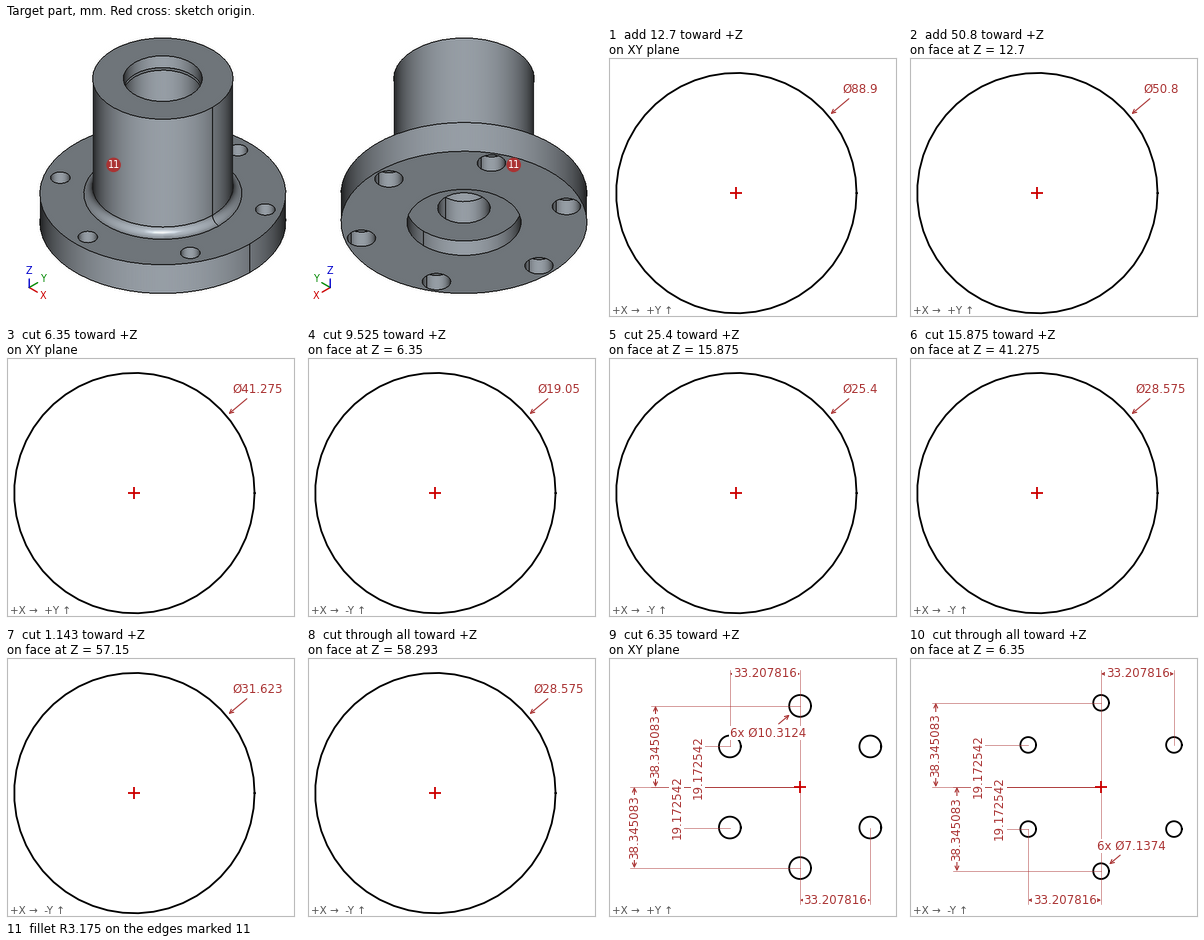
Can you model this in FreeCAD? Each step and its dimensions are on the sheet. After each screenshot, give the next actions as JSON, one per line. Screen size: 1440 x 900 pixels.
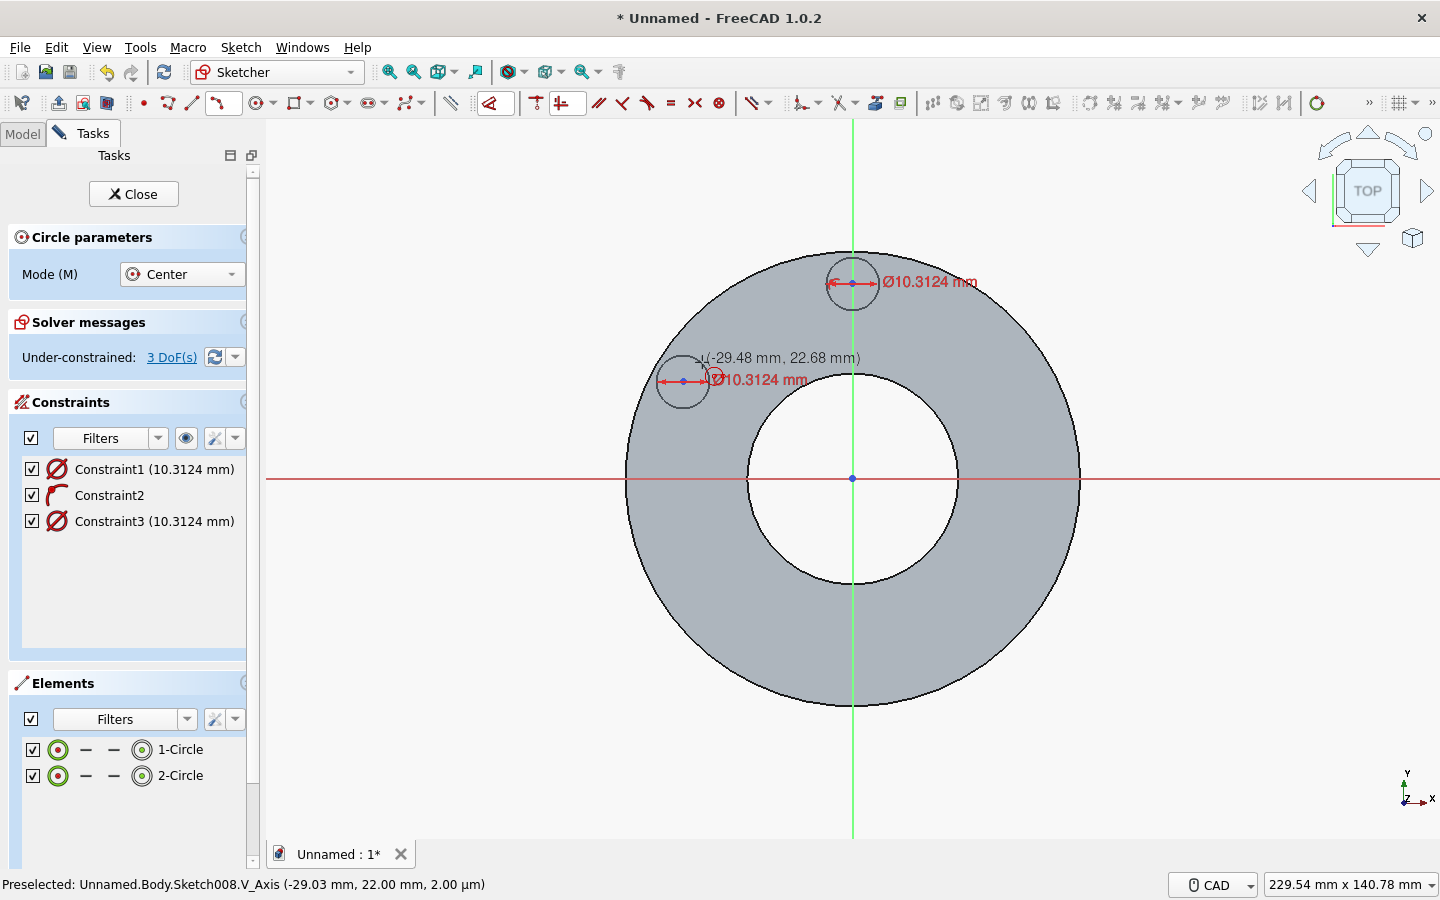
{"action": "left_click", "coordinate": [683, 577]}
{"action": "mouse_move", "coordinate": [702, 558]}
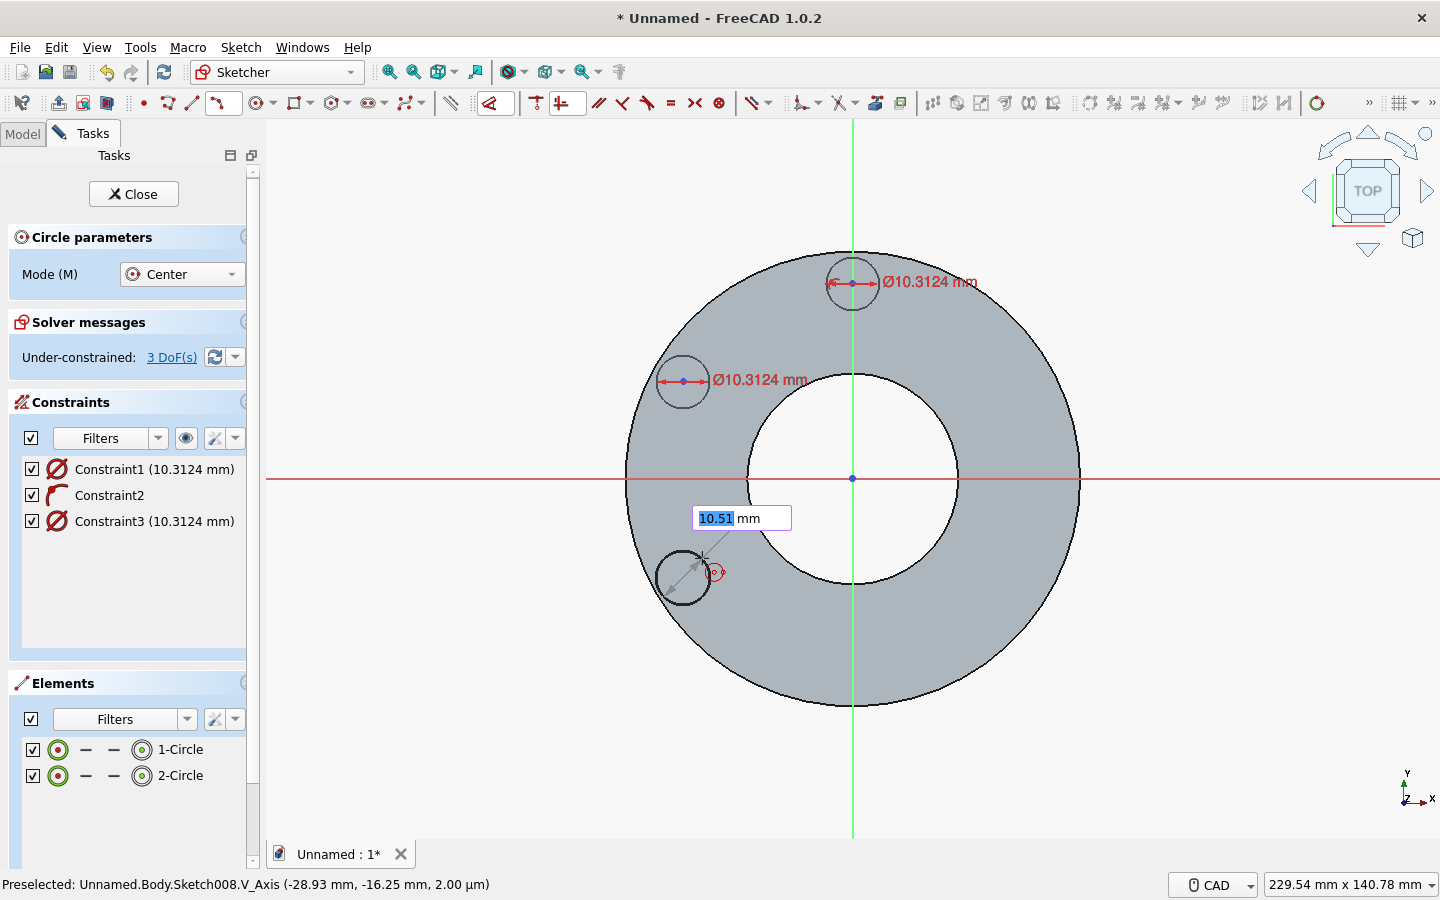
{"action": "type", "text": "10.3124"}
{"action": "key", "text": "Return"}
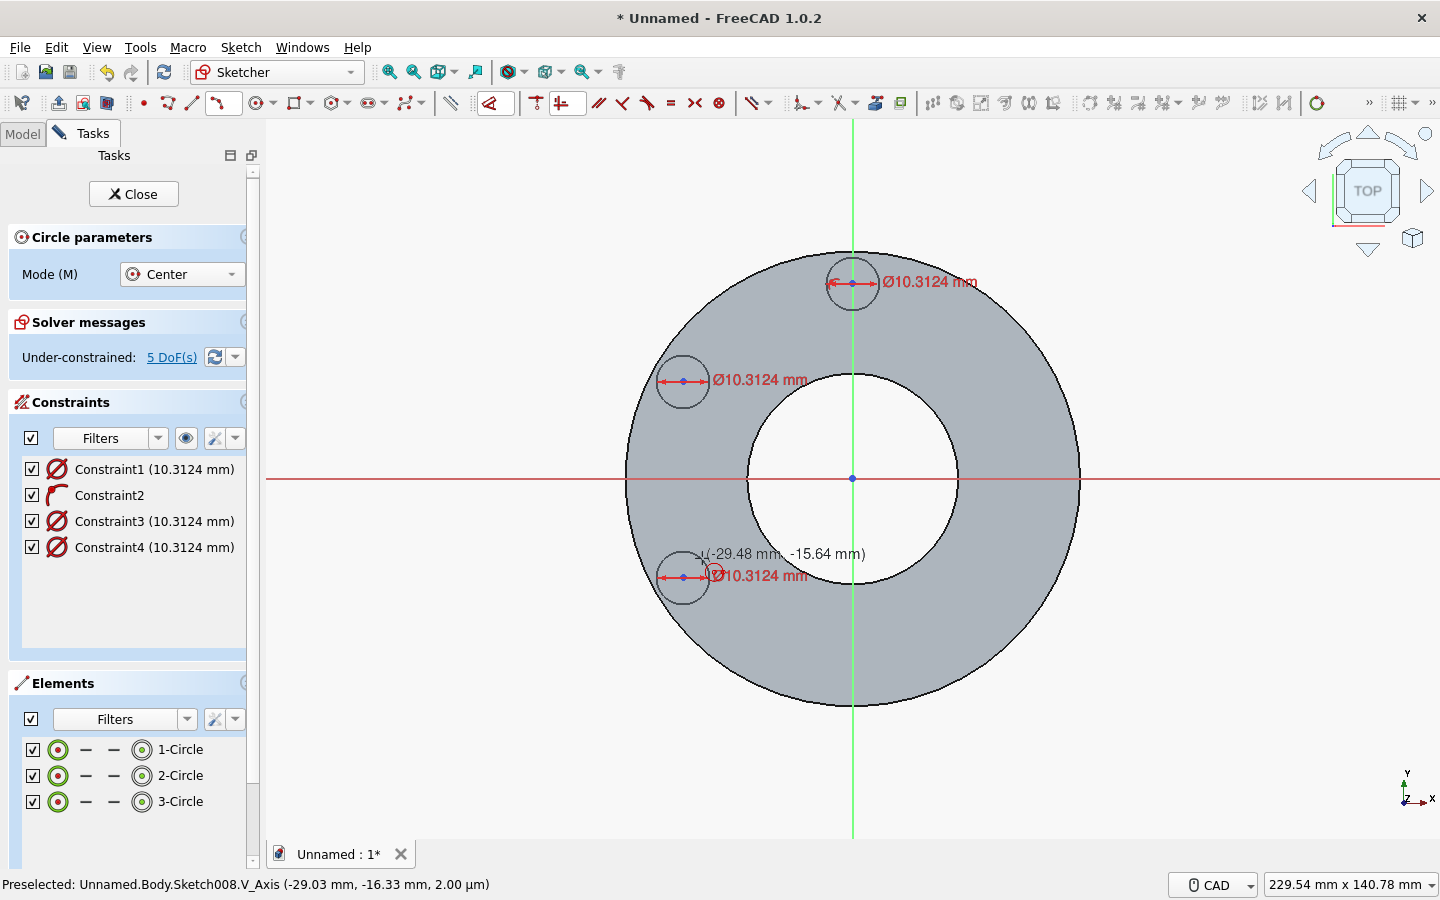
{"action": "left_click", "coordinate": [853, 675]}
{"action": "mouse_move", "coordinate": [871, 656]}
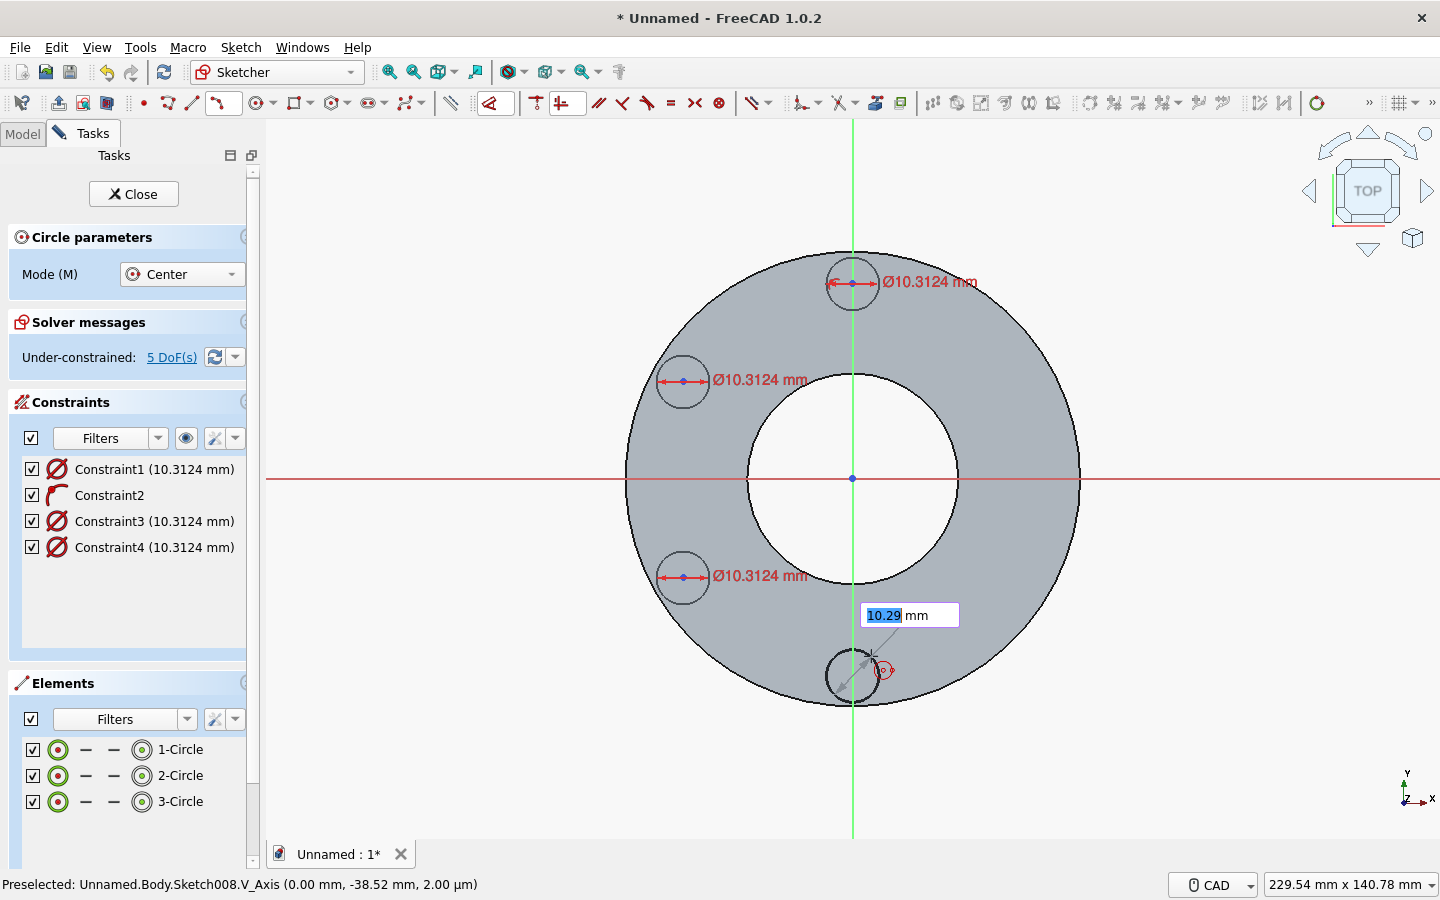
{"action": "type", "text": "10.3124"}
{"action": "key", "text": "Return"}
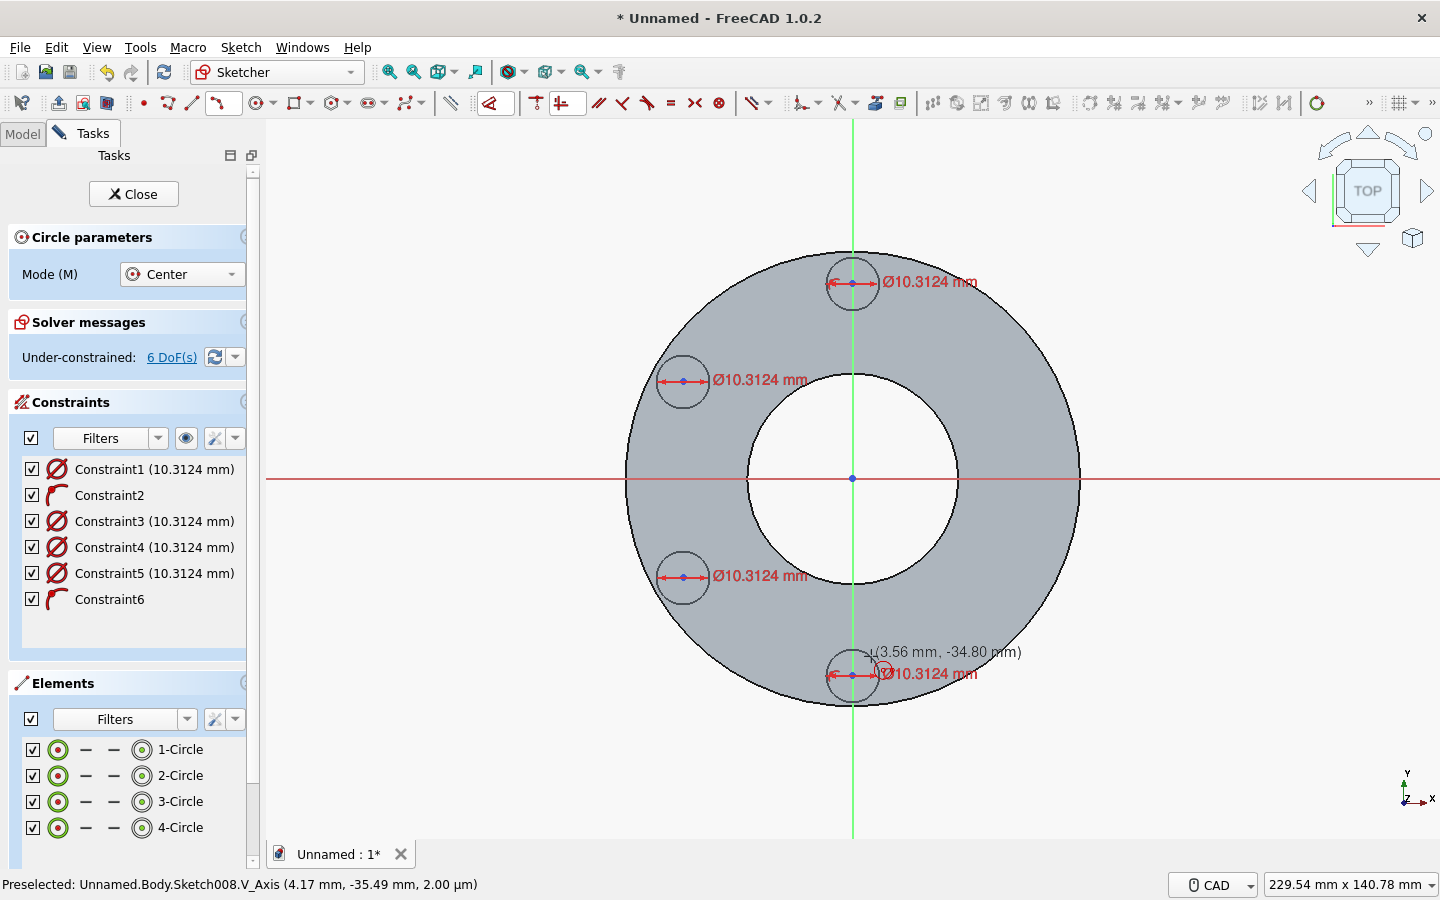
{"action": "left_click", "coordinate": [1023, 577]}
{"action": "mouse_move", "coordinate": [1041, 558]}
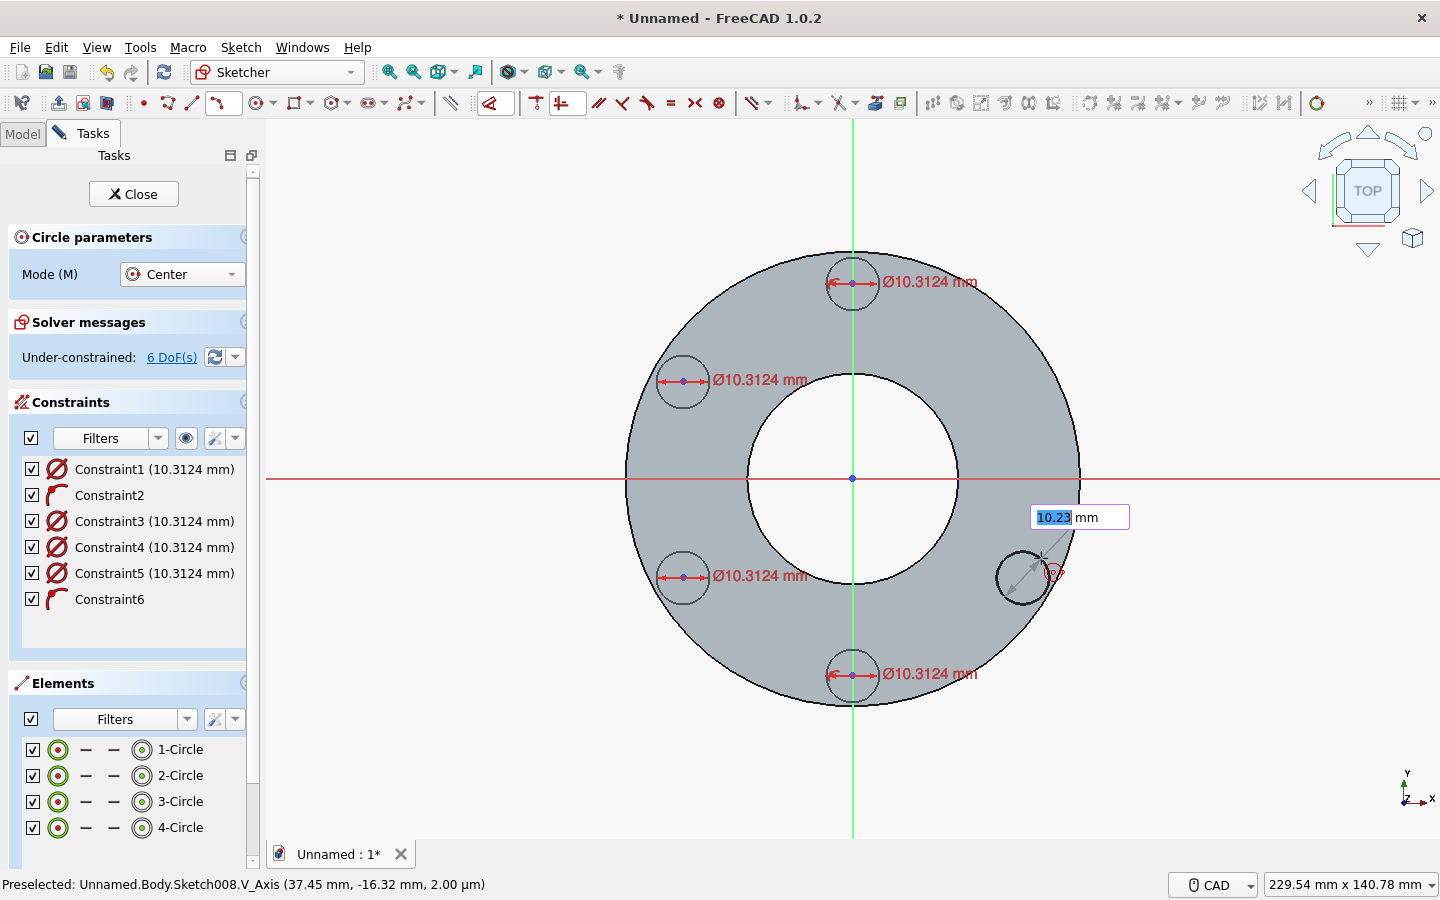
{"action": "type", "text": "10.3124"}
{"action": "key", "text": "Return"}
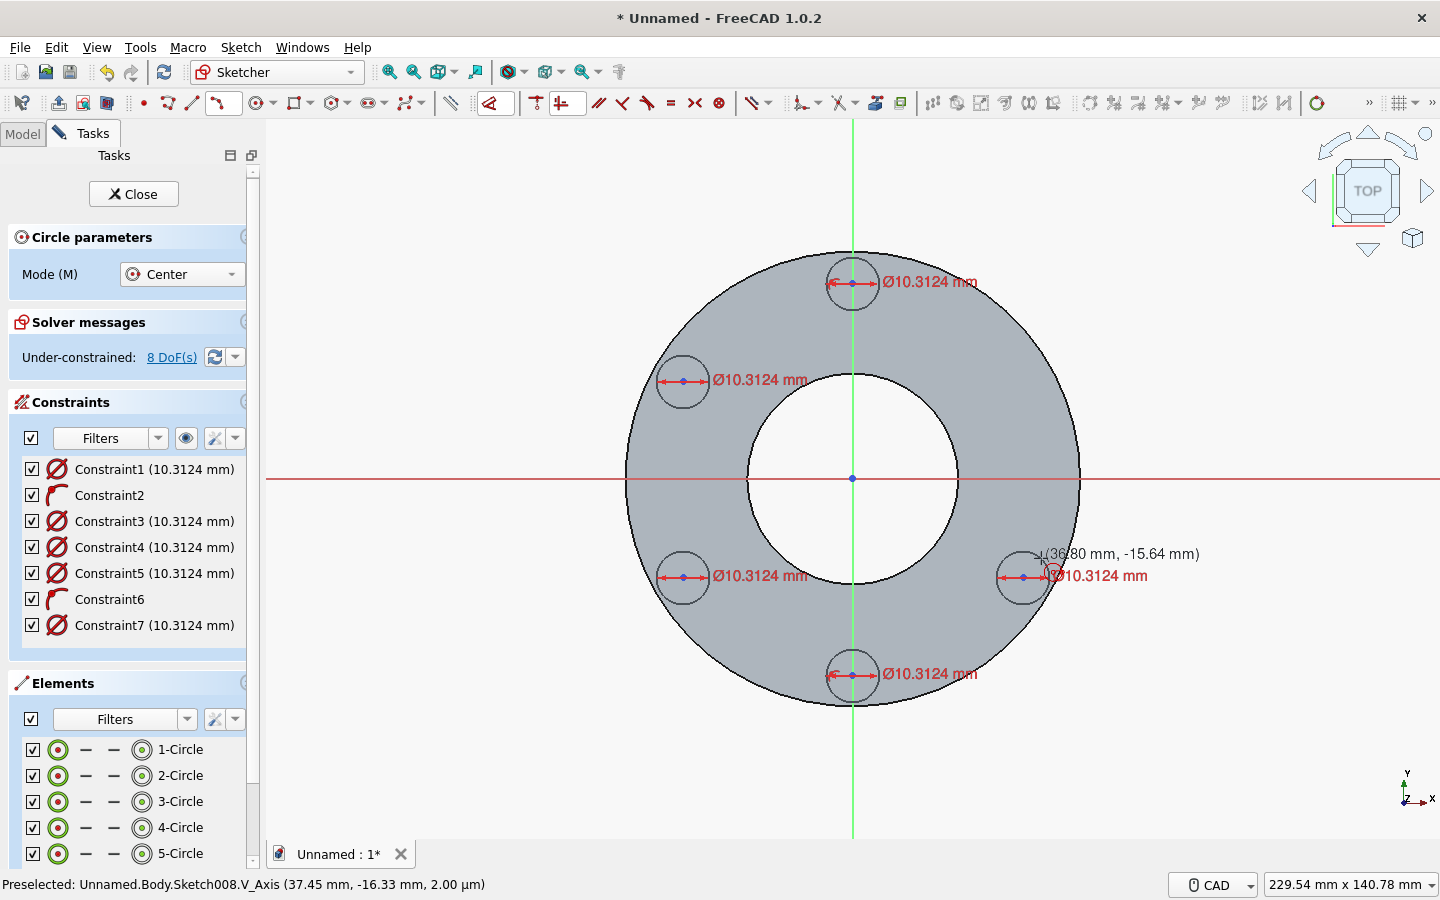
{"action": "left_click", "coordinate": [1023, 381]}
{"action": "mouse_move", "coordinate": [1041, 362]}